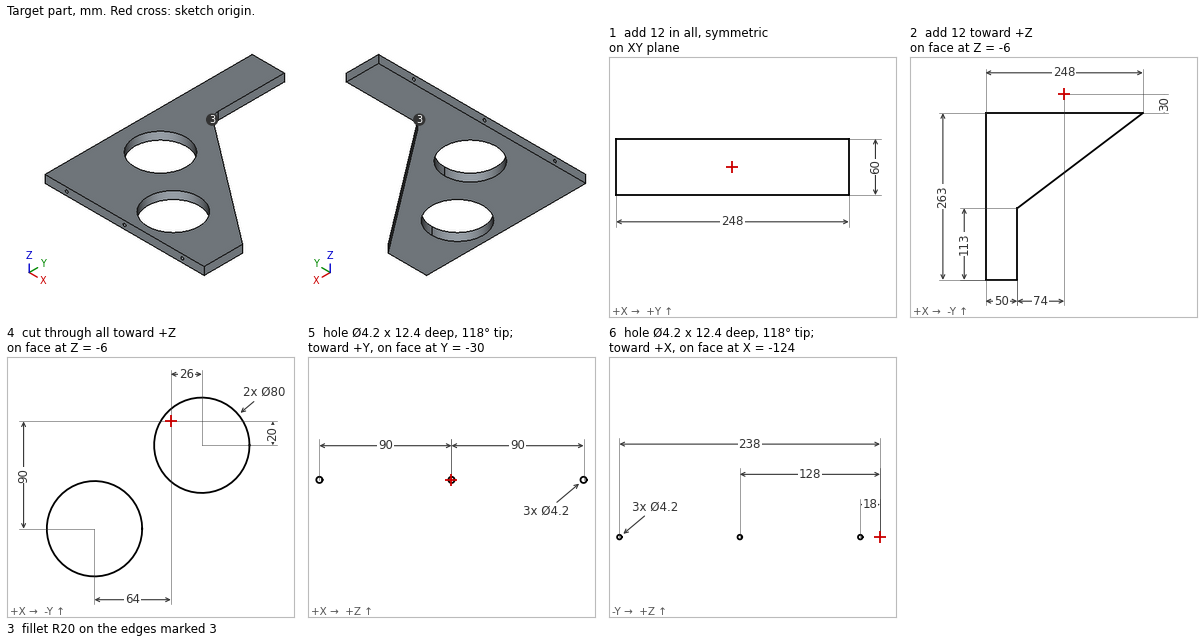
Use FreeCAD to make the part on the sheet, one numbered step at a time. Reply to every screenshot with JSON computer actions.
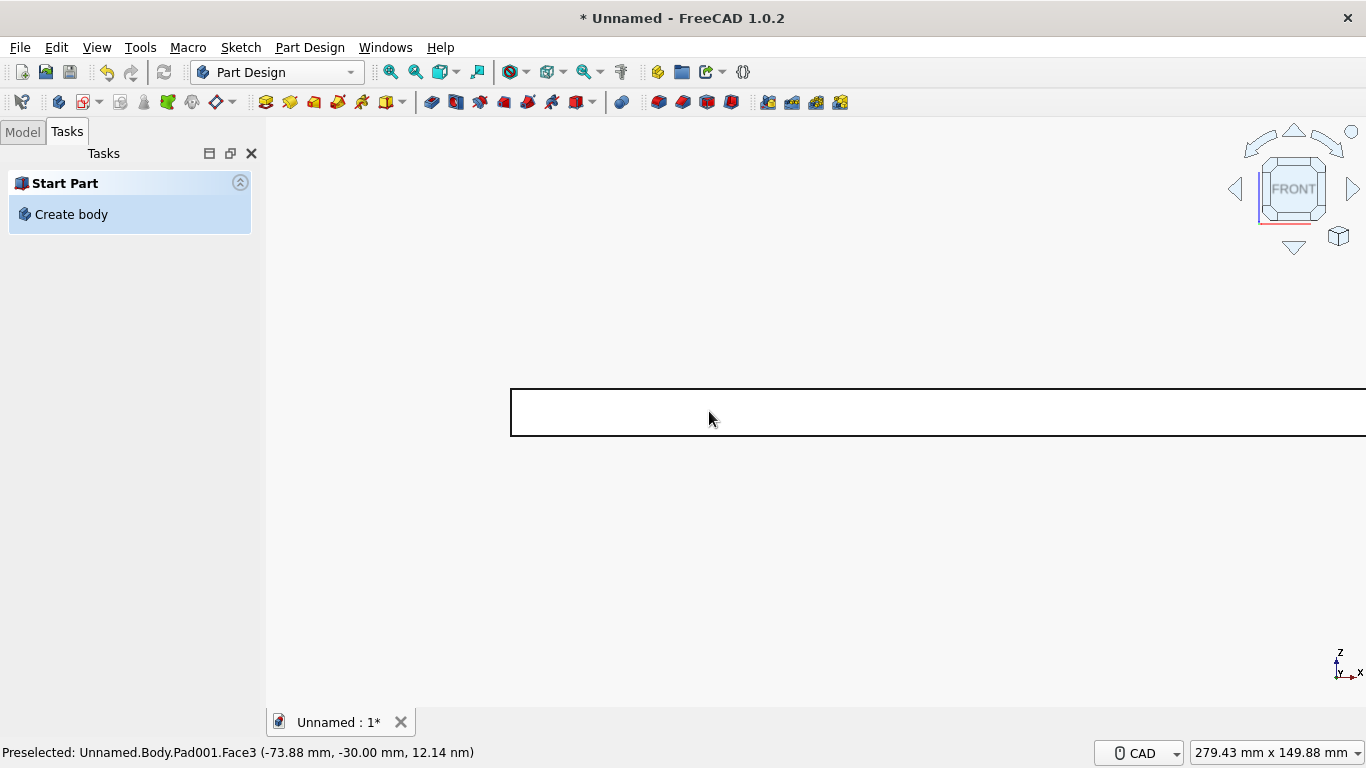
{"action": "key", "text": "v f"}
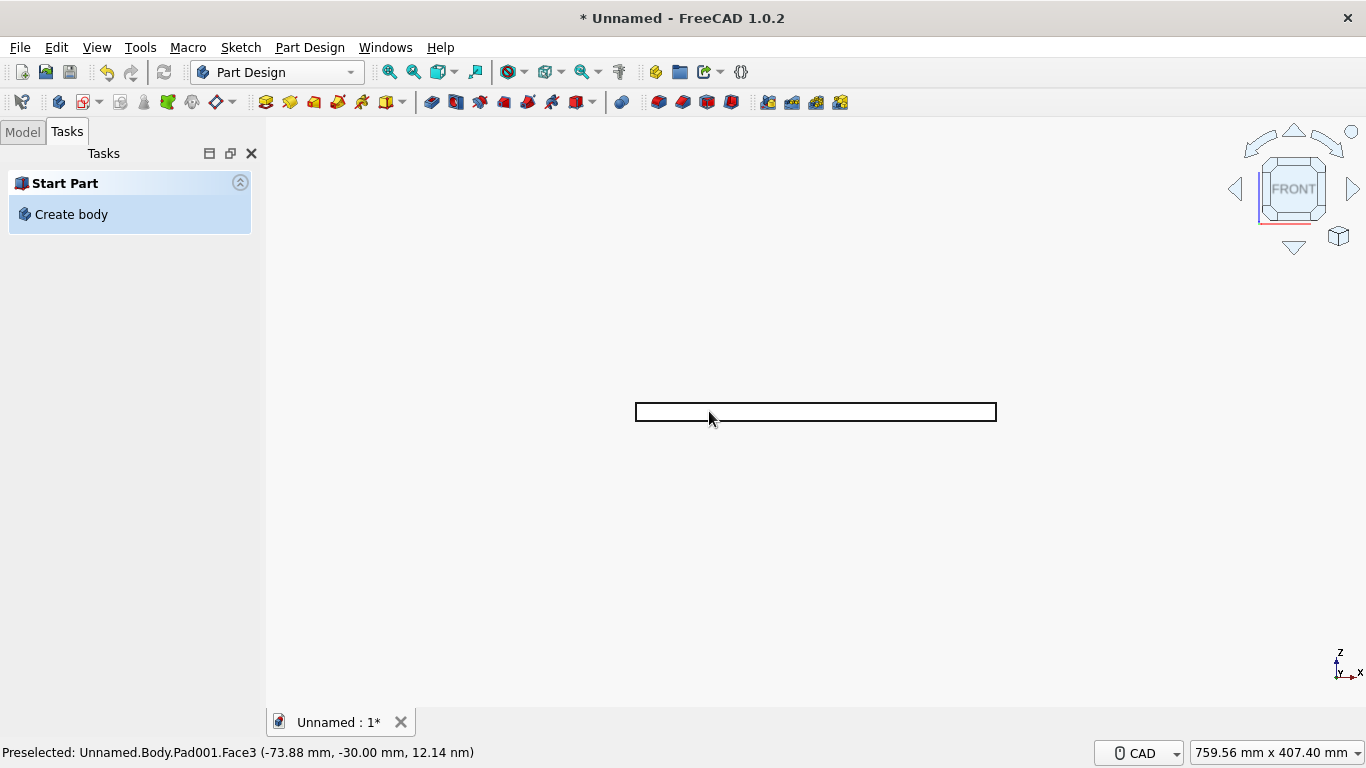
{"action": "key", "text": "3"}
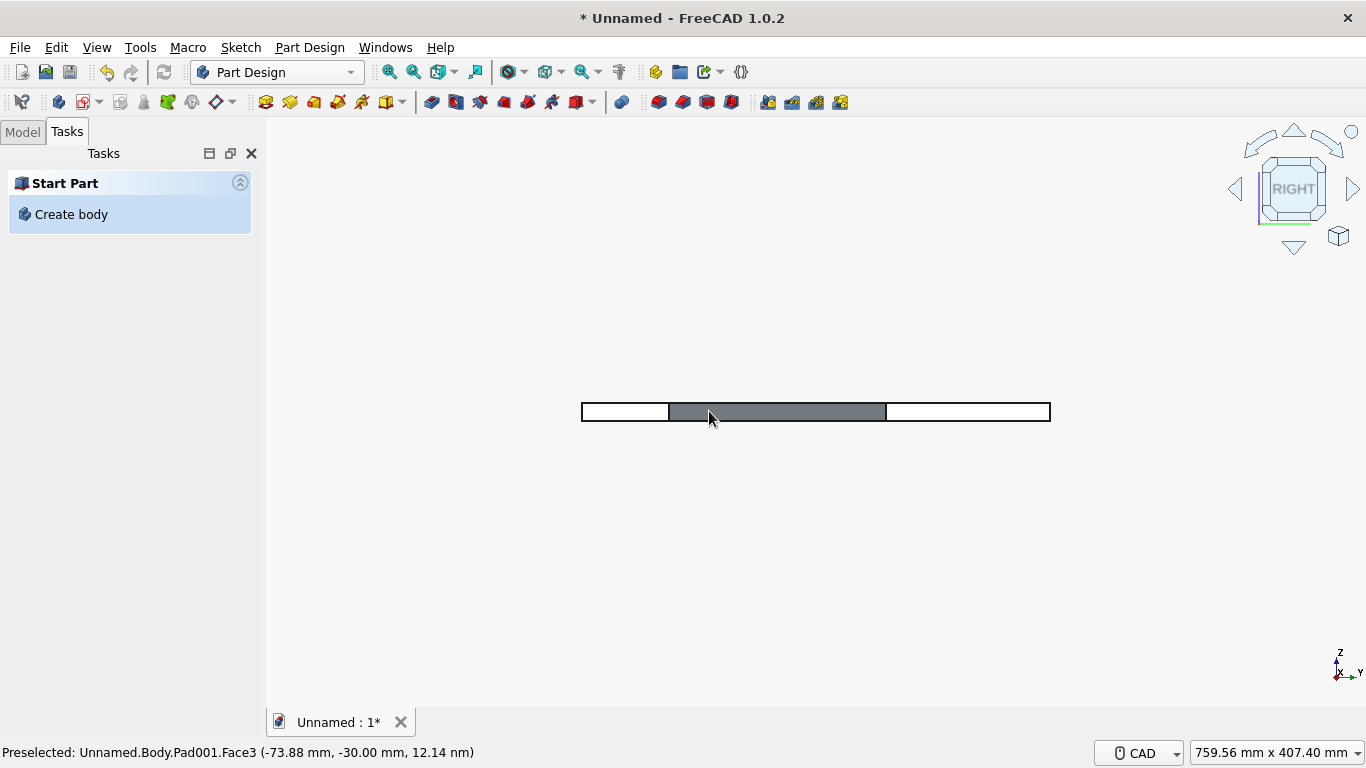
{"action": "key", "text": "v f"}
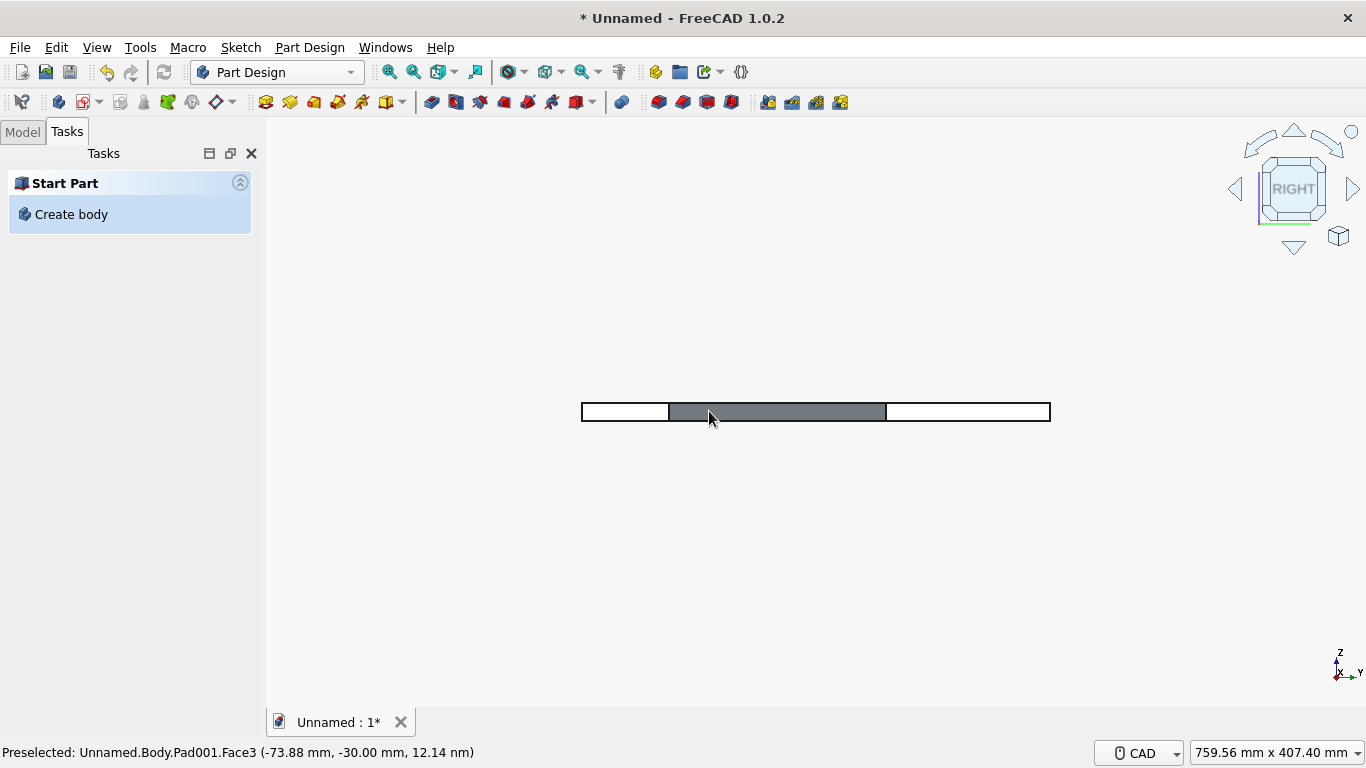
{"action": "scroll", "coordinate": [886, 411], "scroll_direction": "up", "scroll_amount": 5}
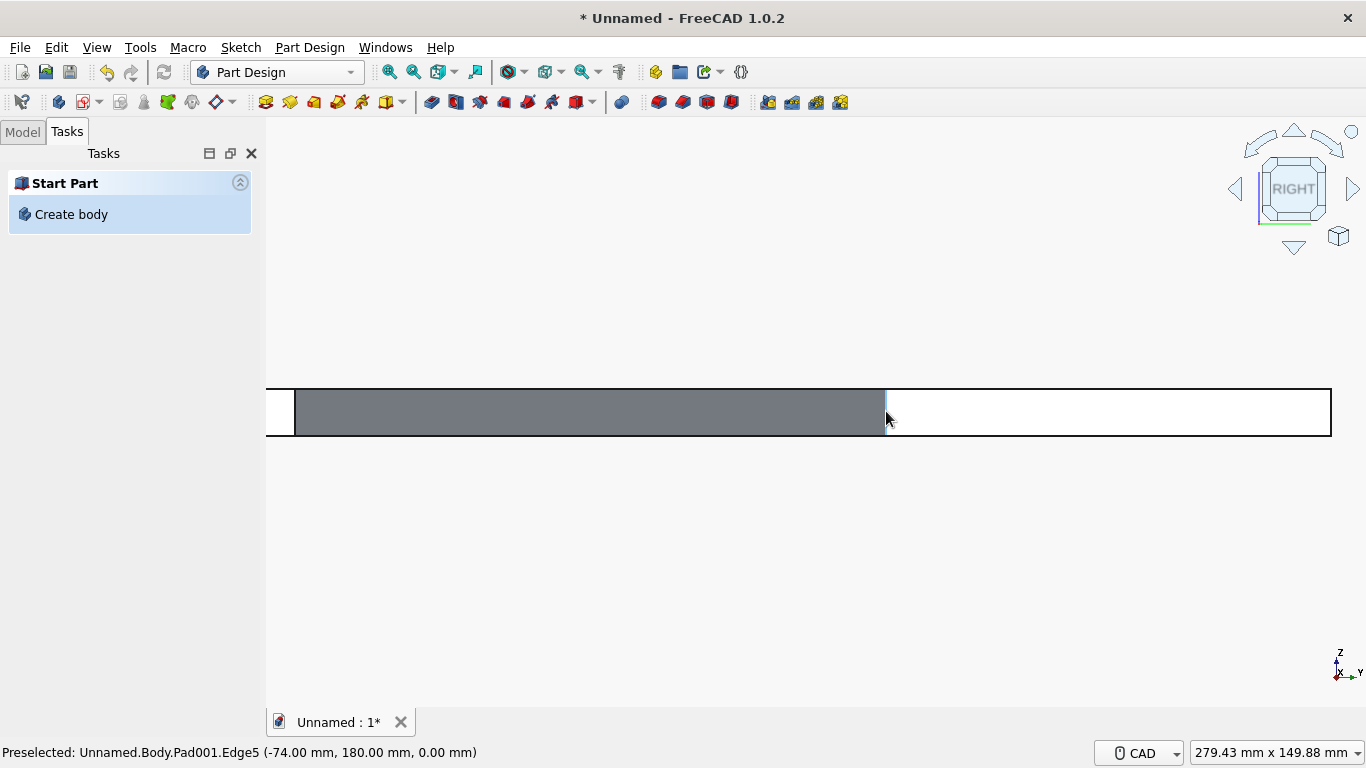
{"action": "left_click", "coordinate": [390, 72]}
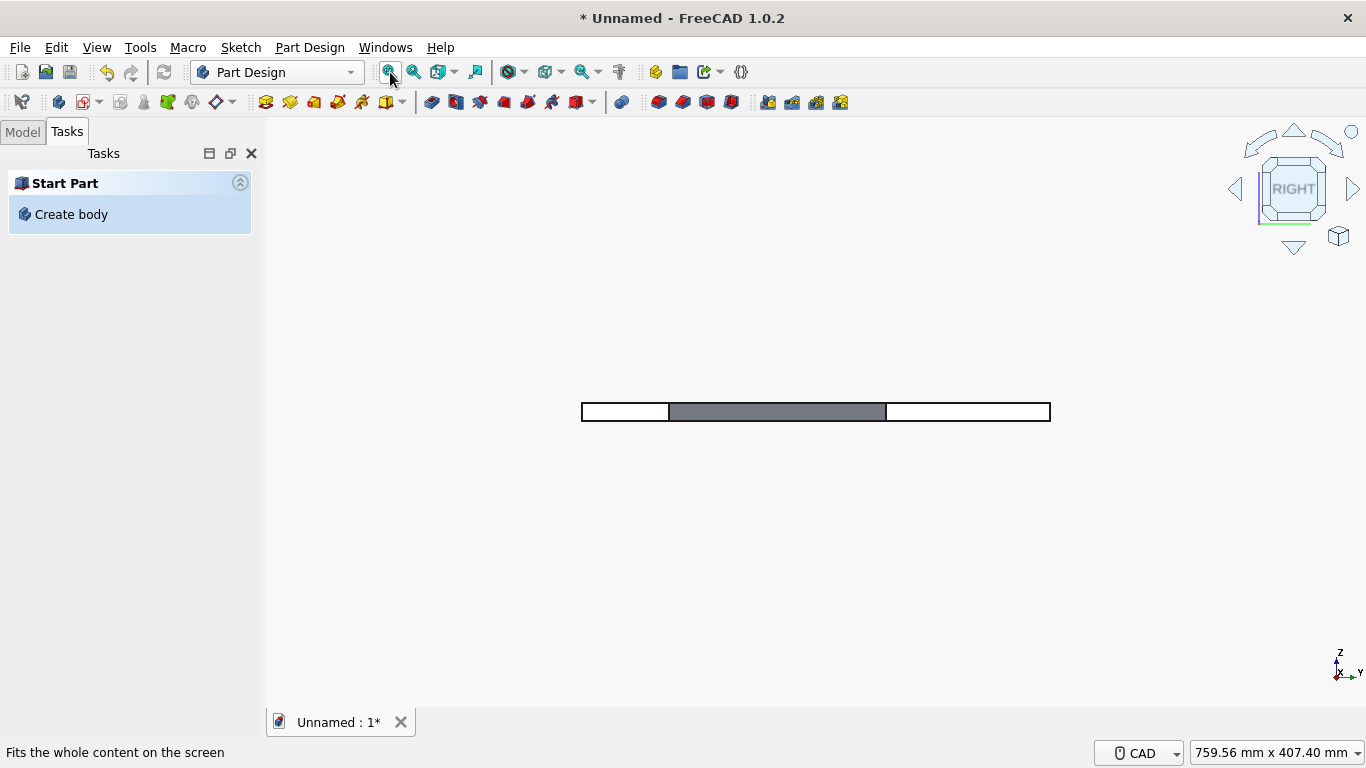
{"action": "key", "text": "5"}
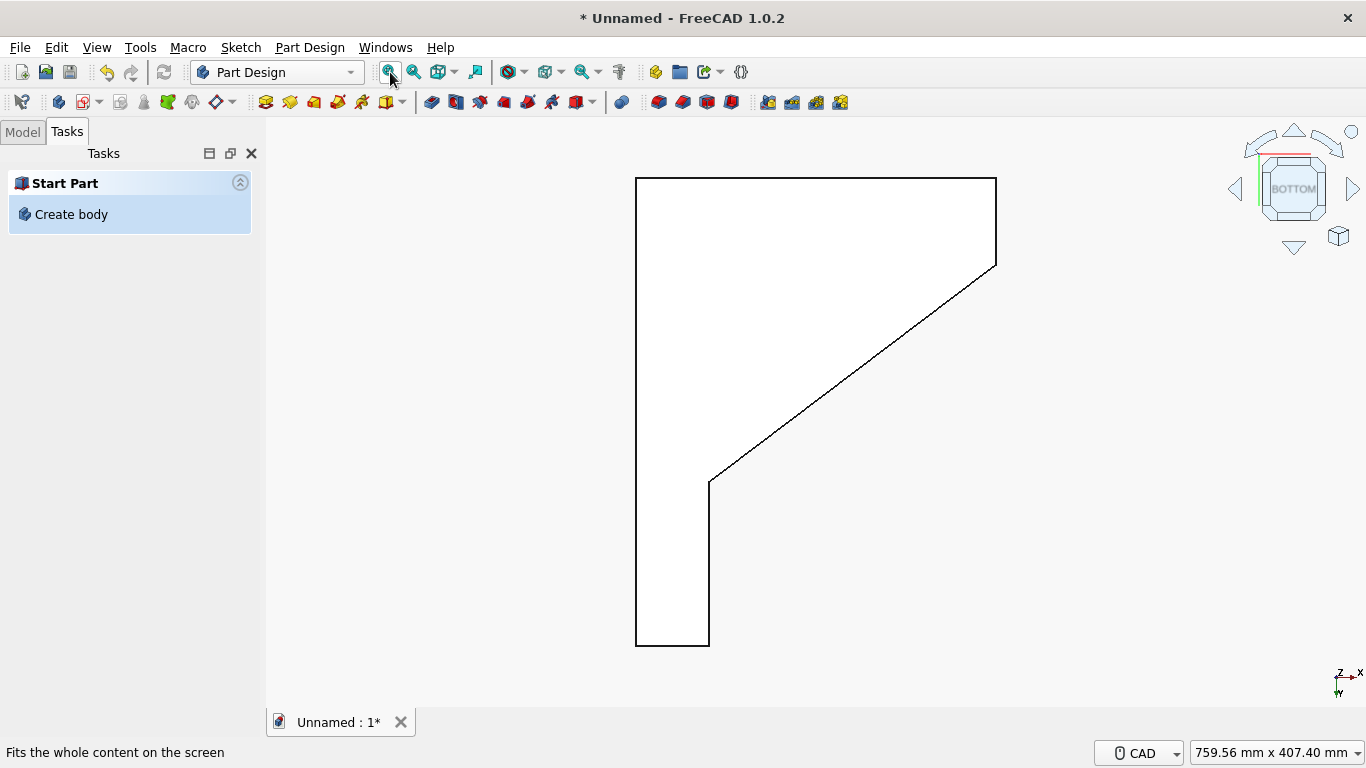
{"action": "scroll", "coordinate": [709, 481], "scroll_direction": "up", "scroll_amount": 5}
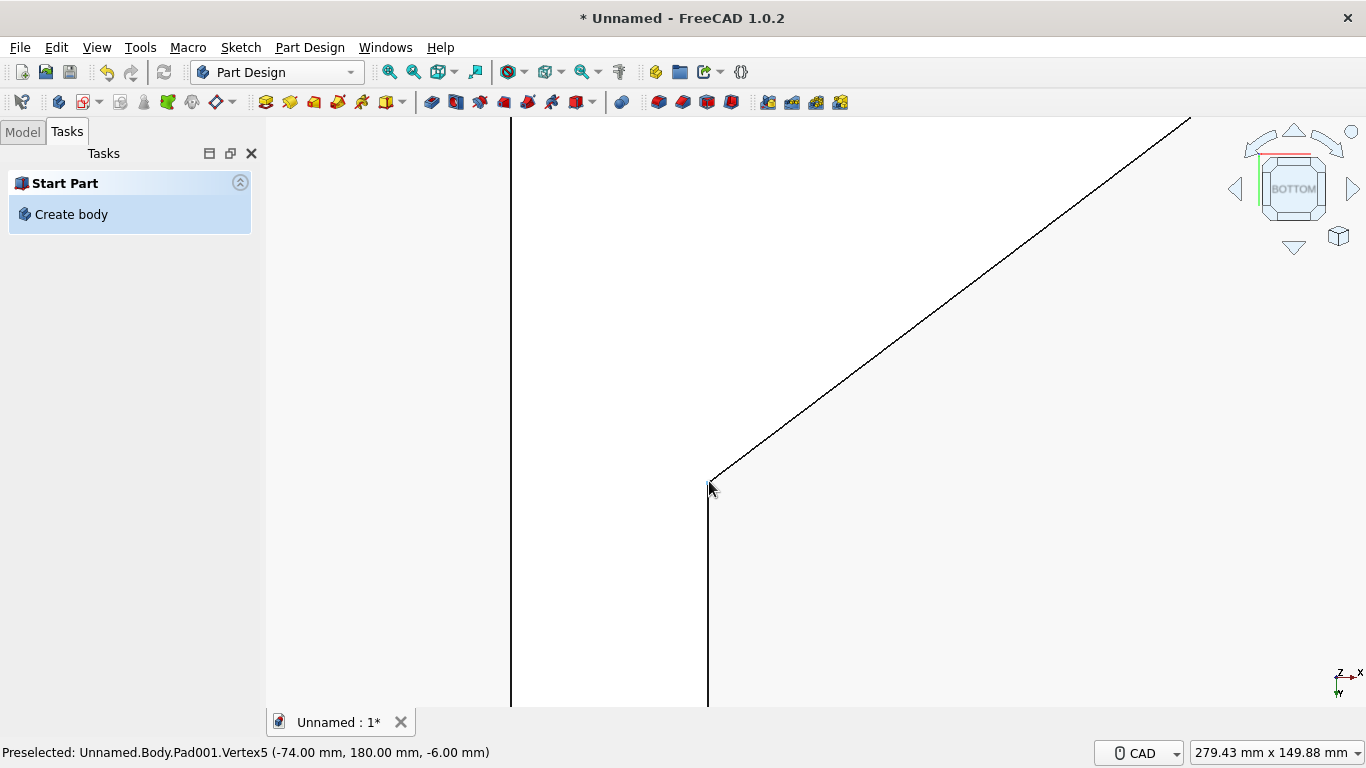
{"action": "left_click", "coordinate": [390, 72]}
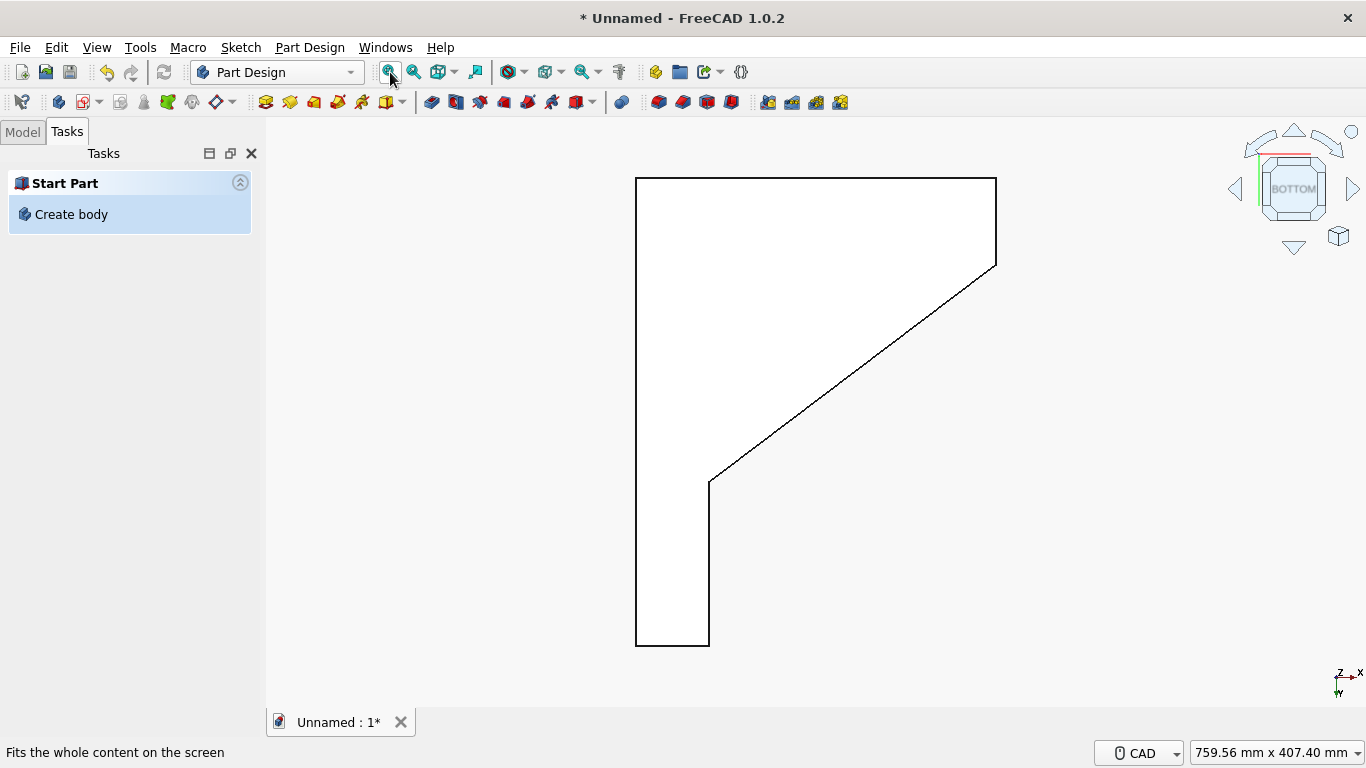
{"action": "key", "text": "4"}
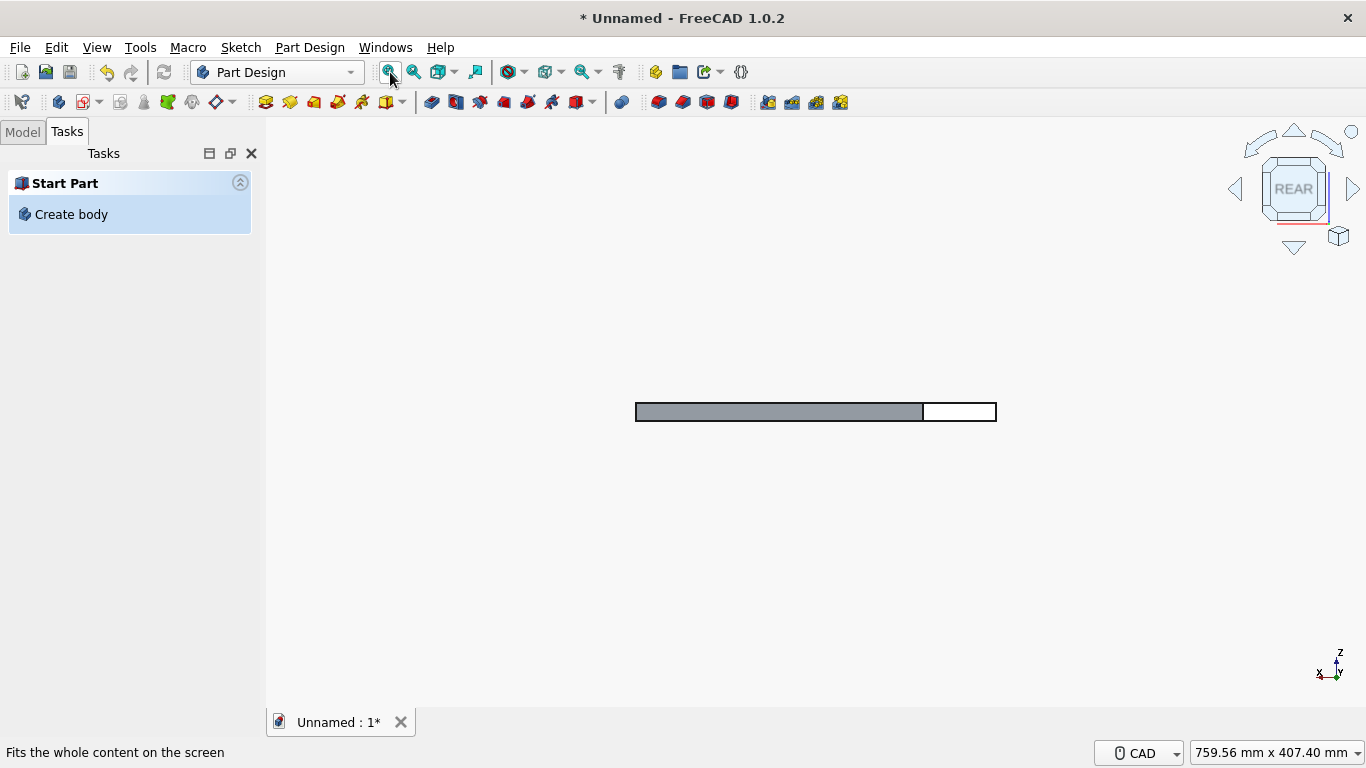
{"action": "key", "text": "v f"}